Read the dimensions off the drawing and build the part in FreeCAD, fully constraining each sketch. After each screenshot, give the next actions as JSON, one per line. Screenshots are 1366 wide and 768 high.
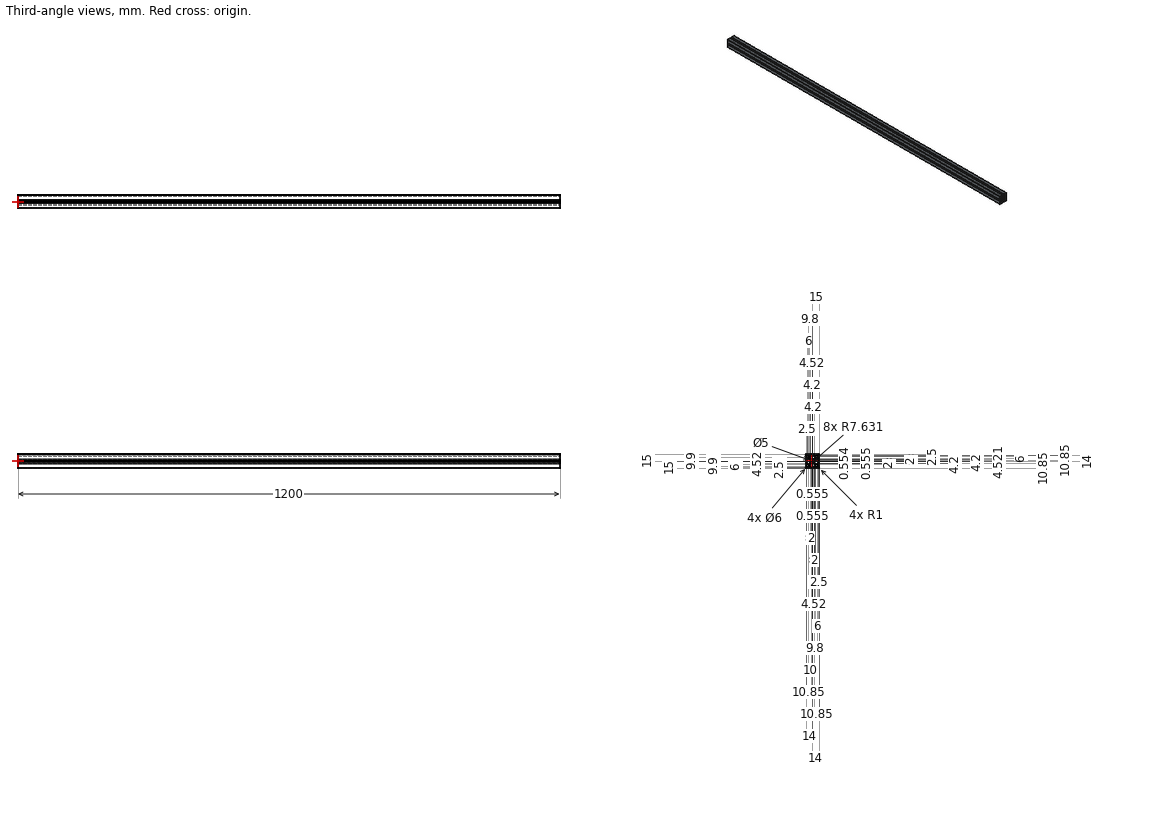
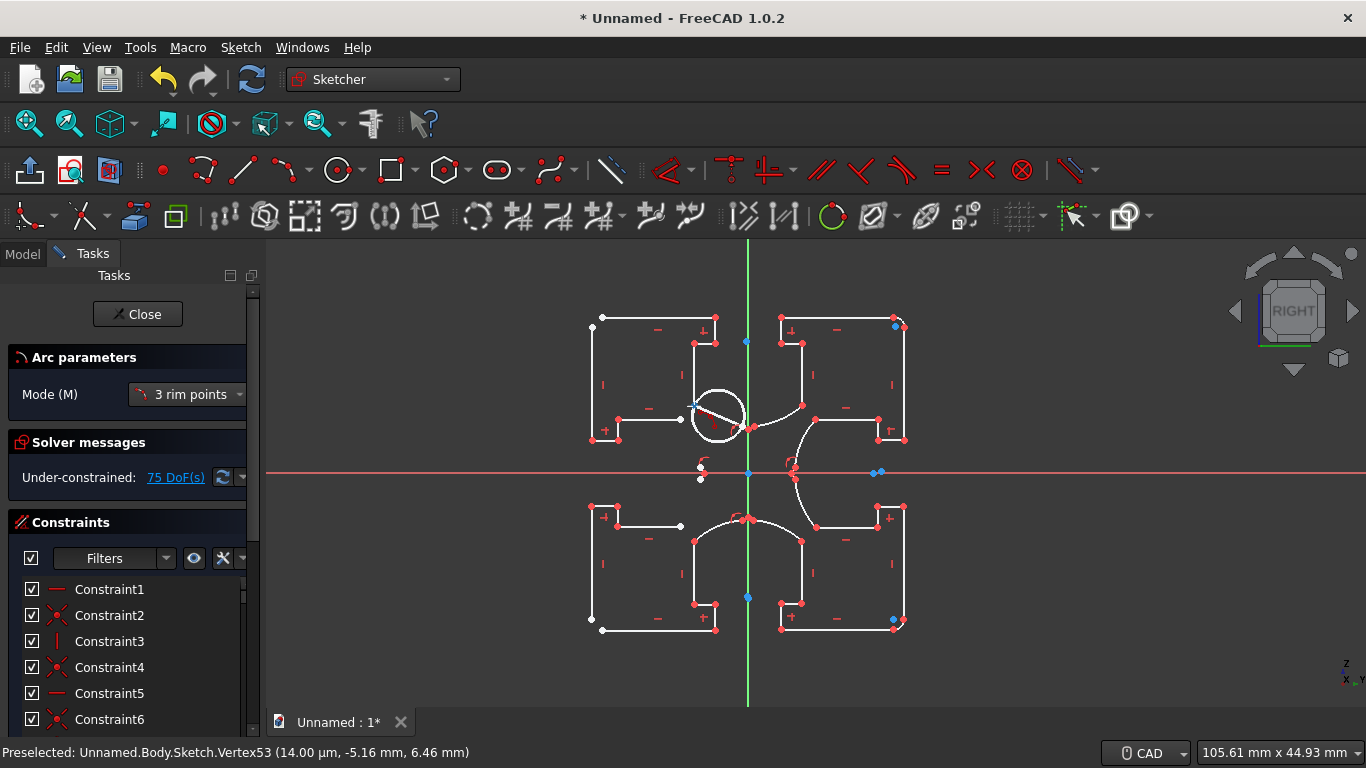
{"action": "scroll", "coordinate": [717, 420], "scroll_direction": "up", "scroll_amount": 7}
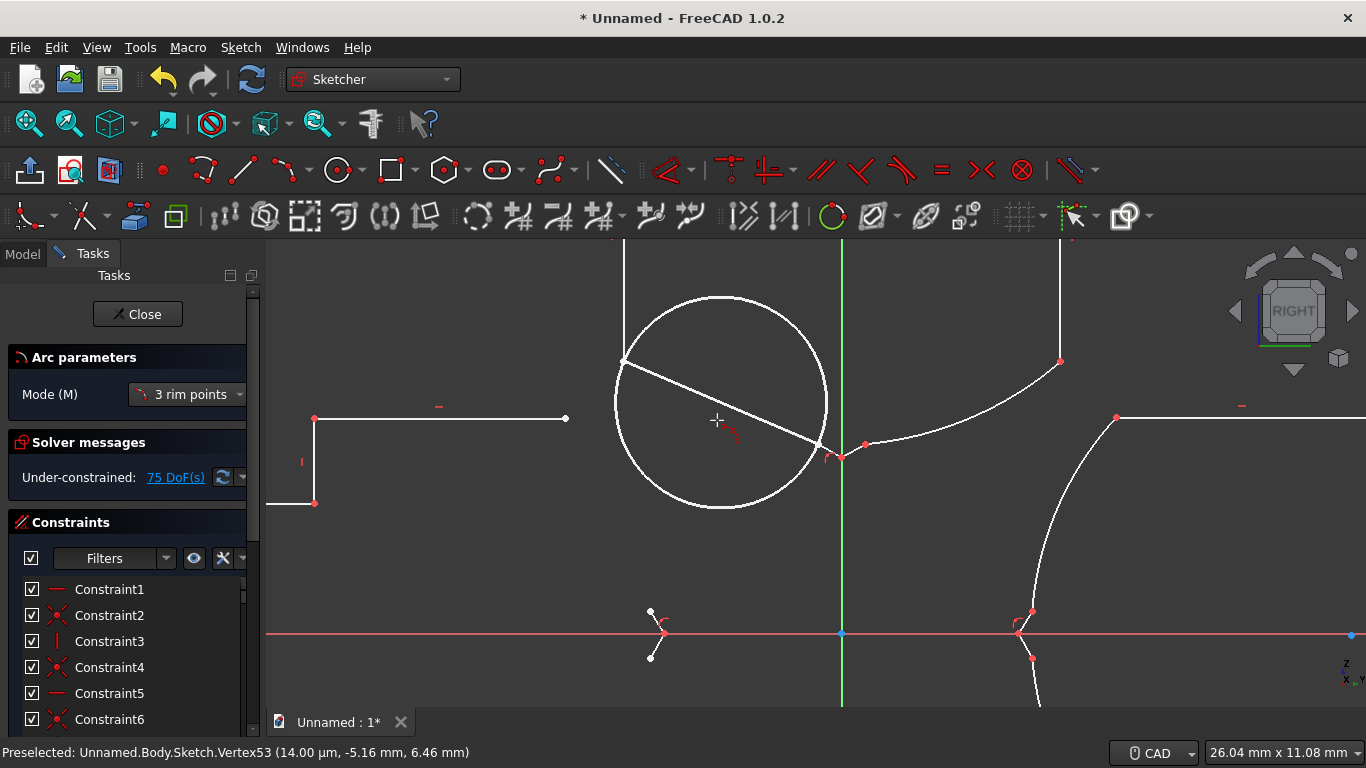
{"action": "left_click", "coordinate": [714, 418]}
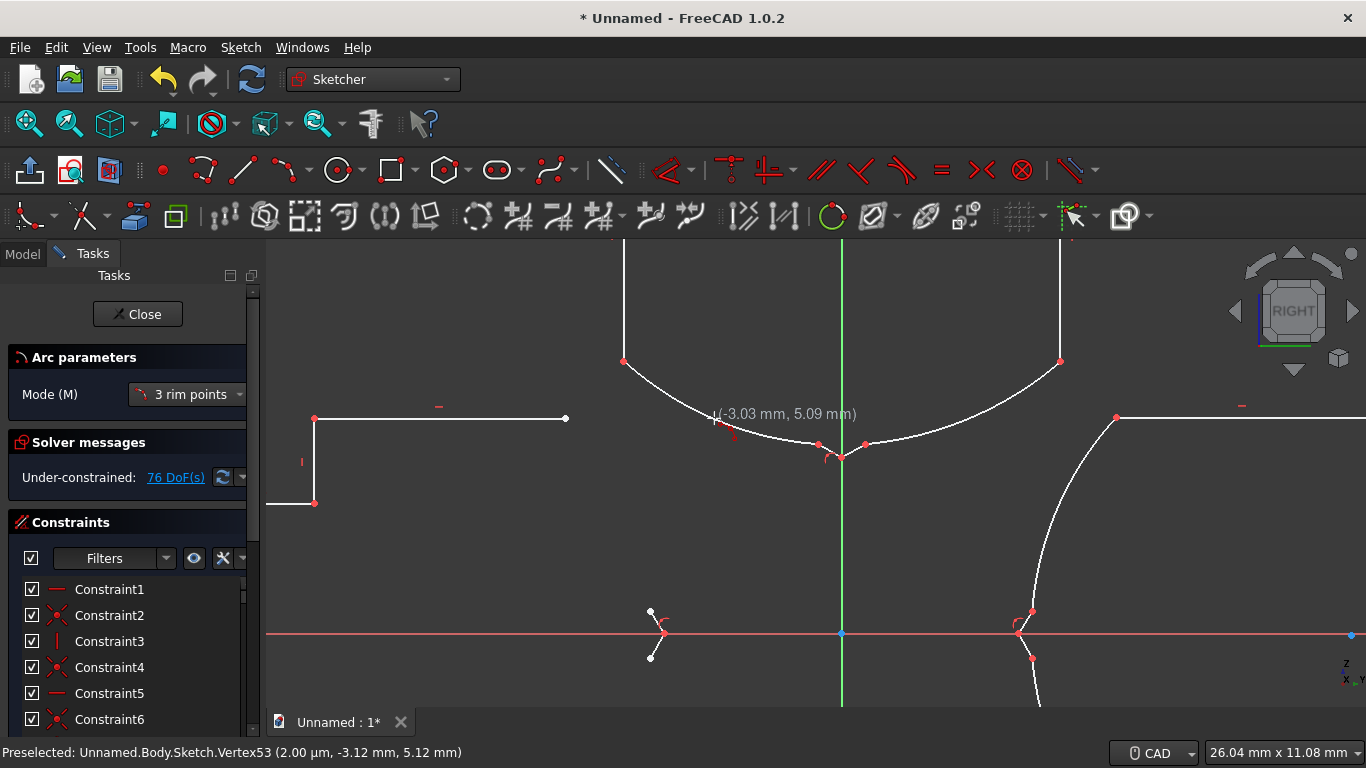
{"action": "scroll", "coordinate": [717, 420], "scroll_direction": "down", "scroll_amount": 7}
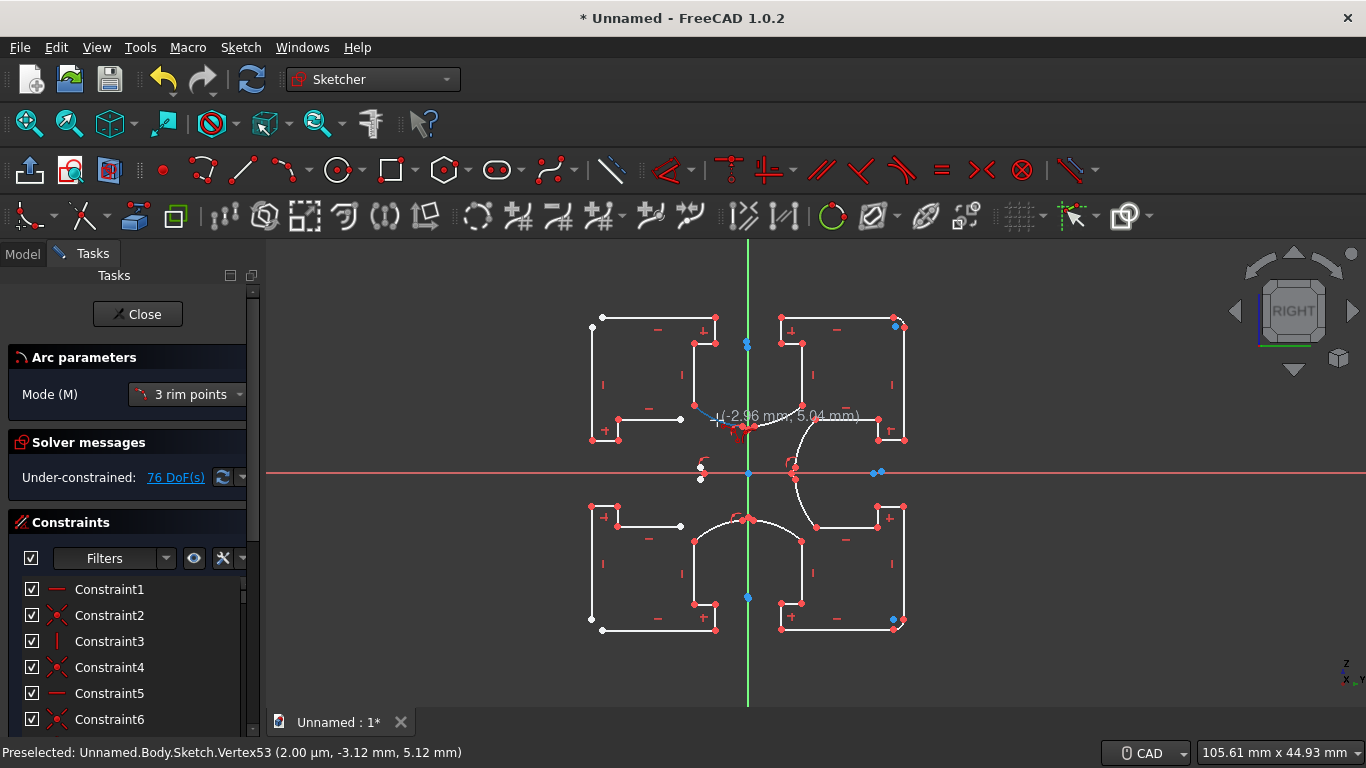
{"action": "left_click", "coordinate": [602, 318]}
{"action": "left_click", "coordinate": [592, 328]}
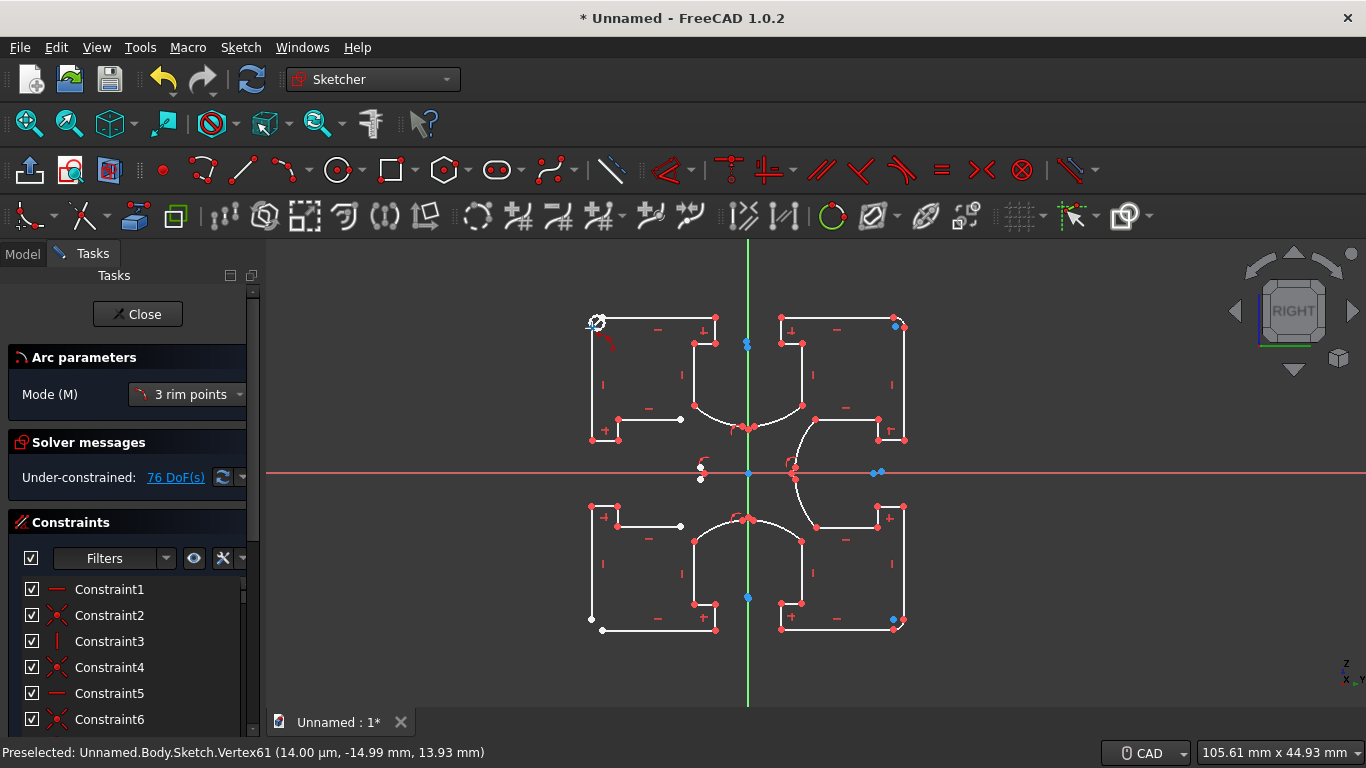
{"action": "scroll", "coordinate": [595, 320], "scroll_direction": "up", "scroll_amount": 9}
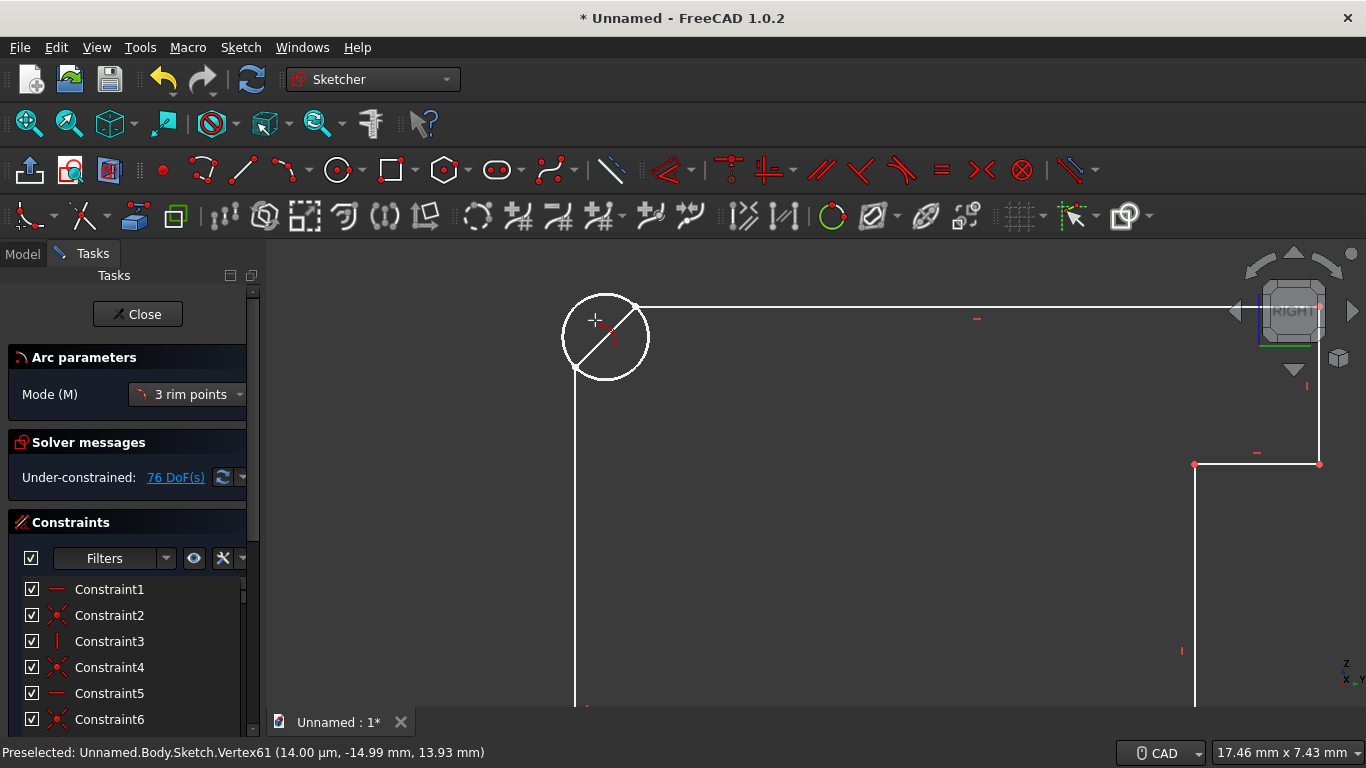
{"action": "left_click", "coordinate": [593, 318]}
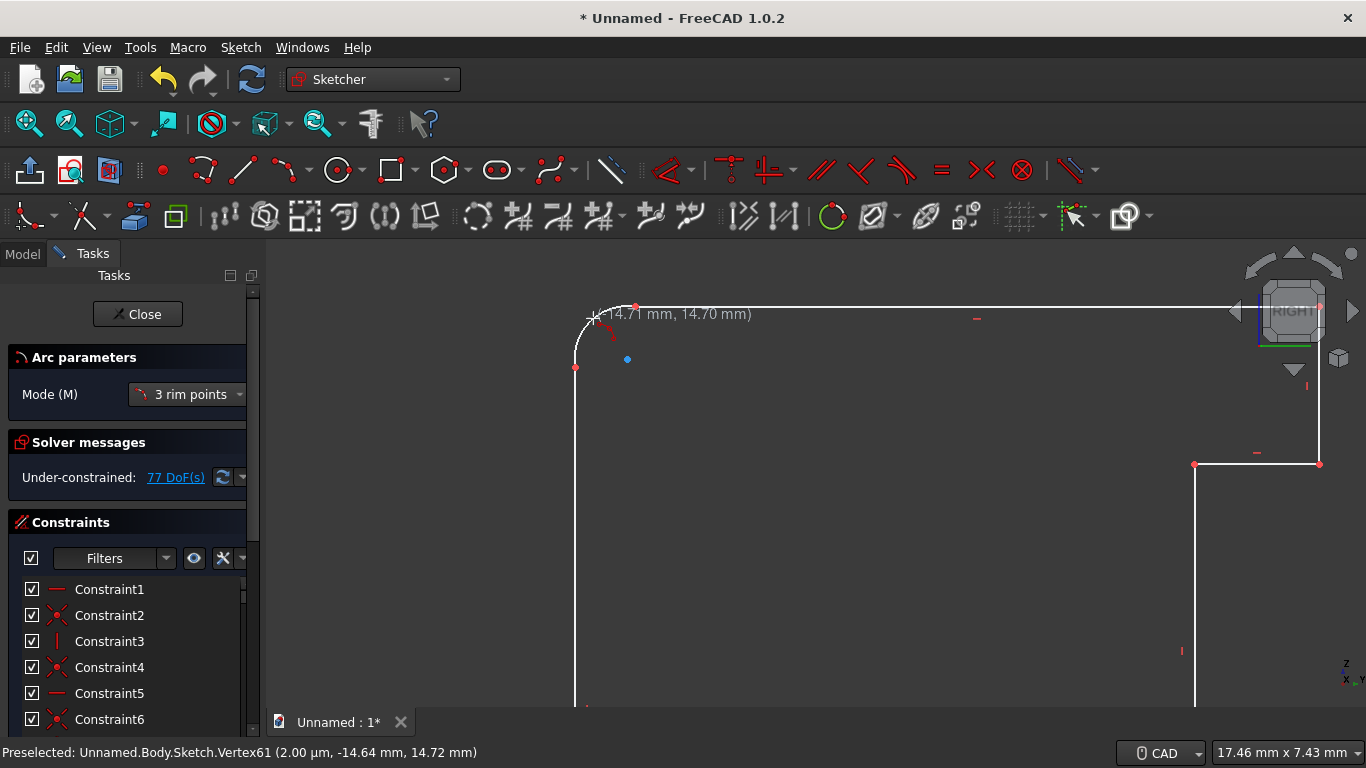
{"action": "scroll", "coordinate": [595, 320], "scroll_direction": "down", "scroll_amount": 9}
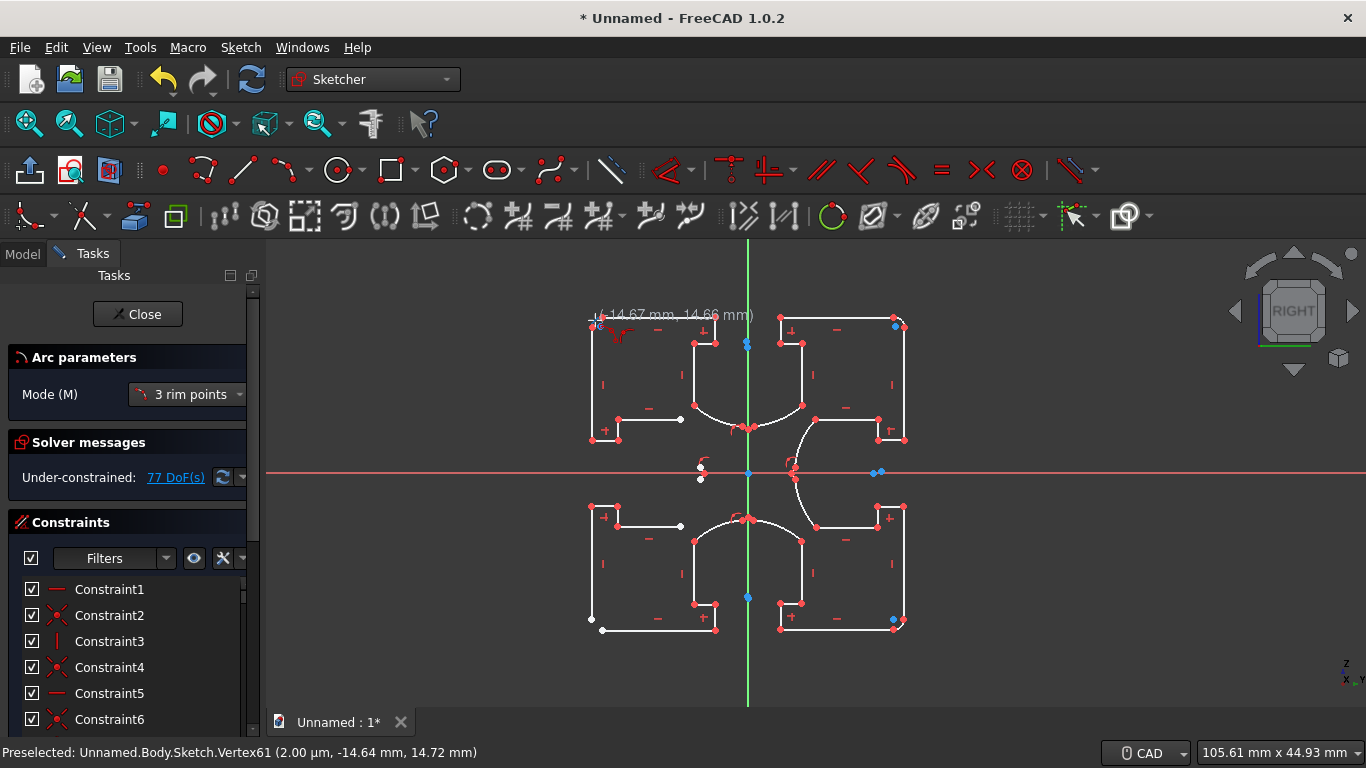
{"action": "left_click", "coordinate": [680, 420]}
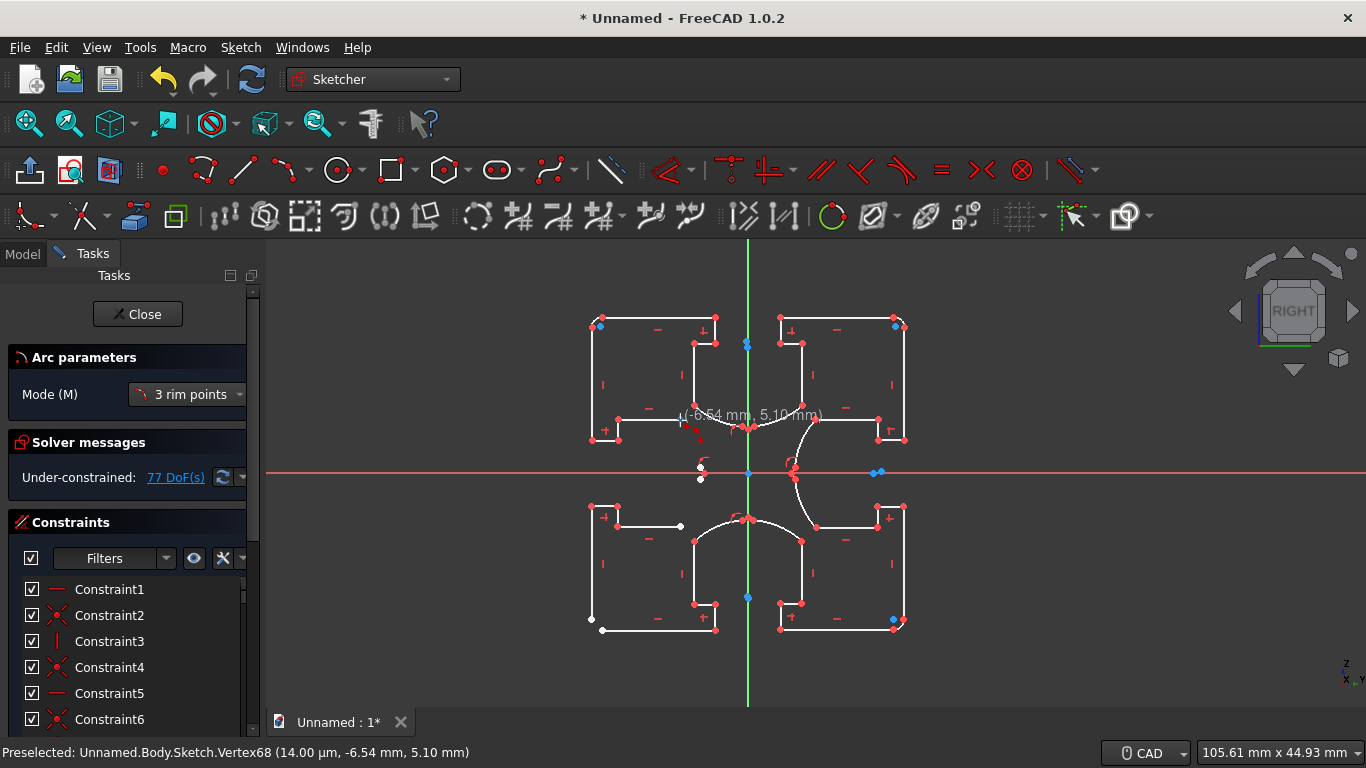
{"action": "scroll", "coordinate": [701, 467], "scroll_direction": "up", "scroll_amount": 8}